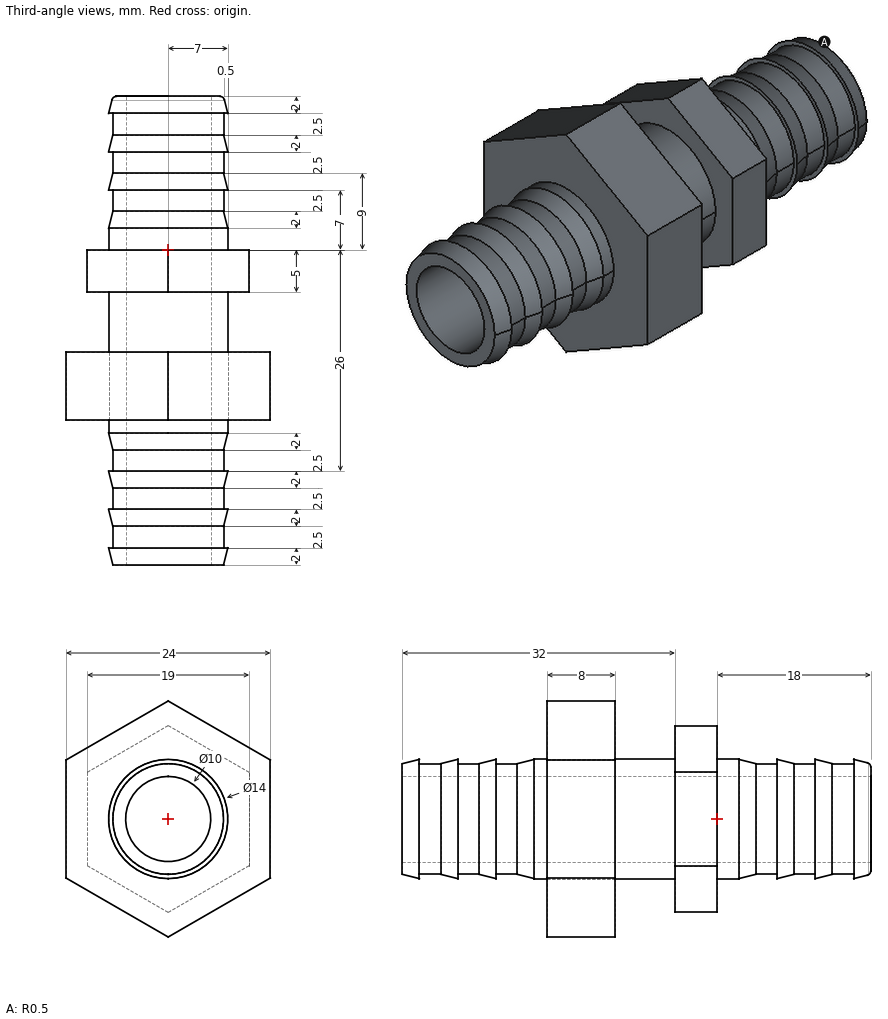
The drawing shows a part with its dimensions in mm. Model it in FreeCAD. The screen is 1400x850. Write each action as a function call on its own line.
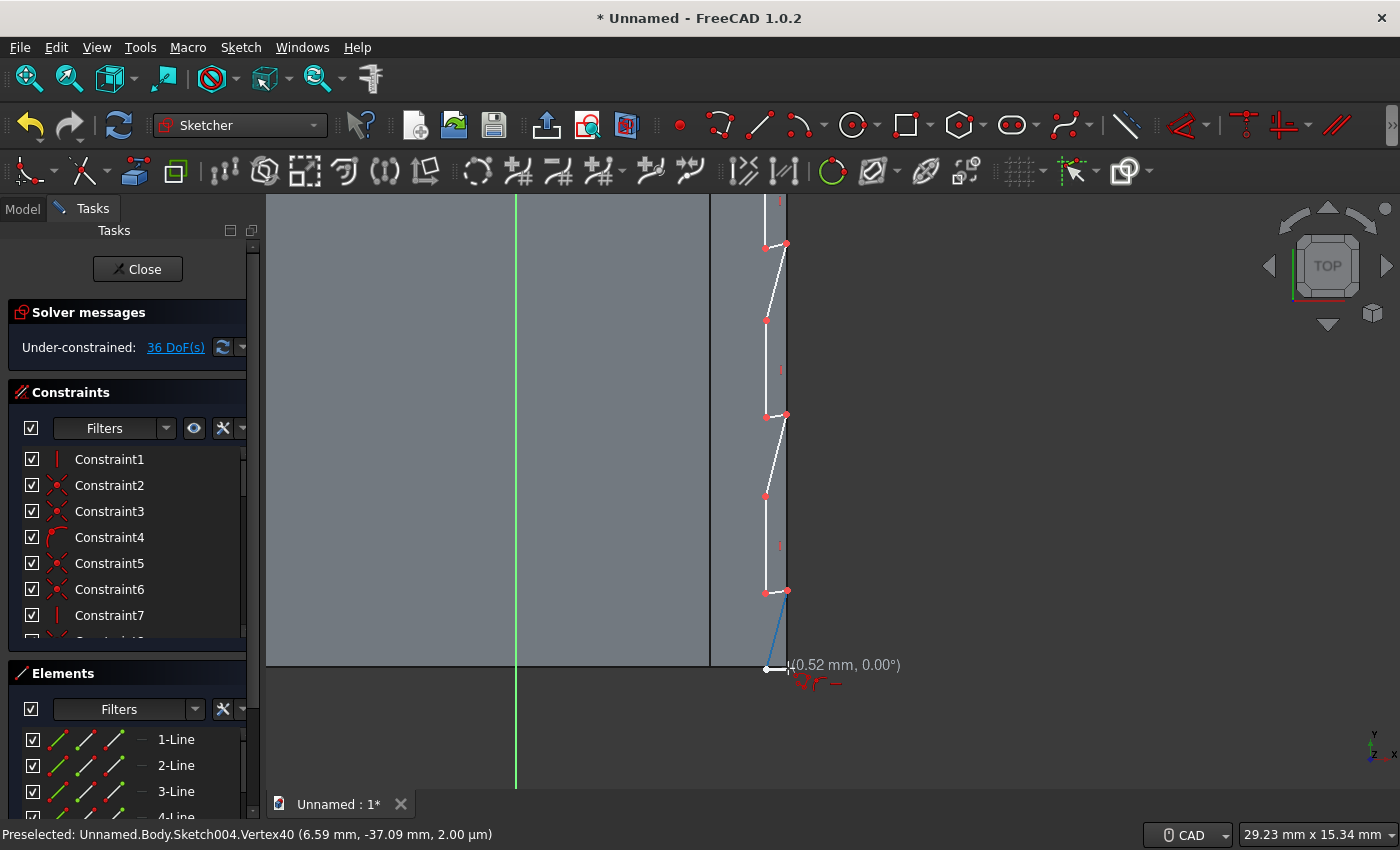
click(787, 666)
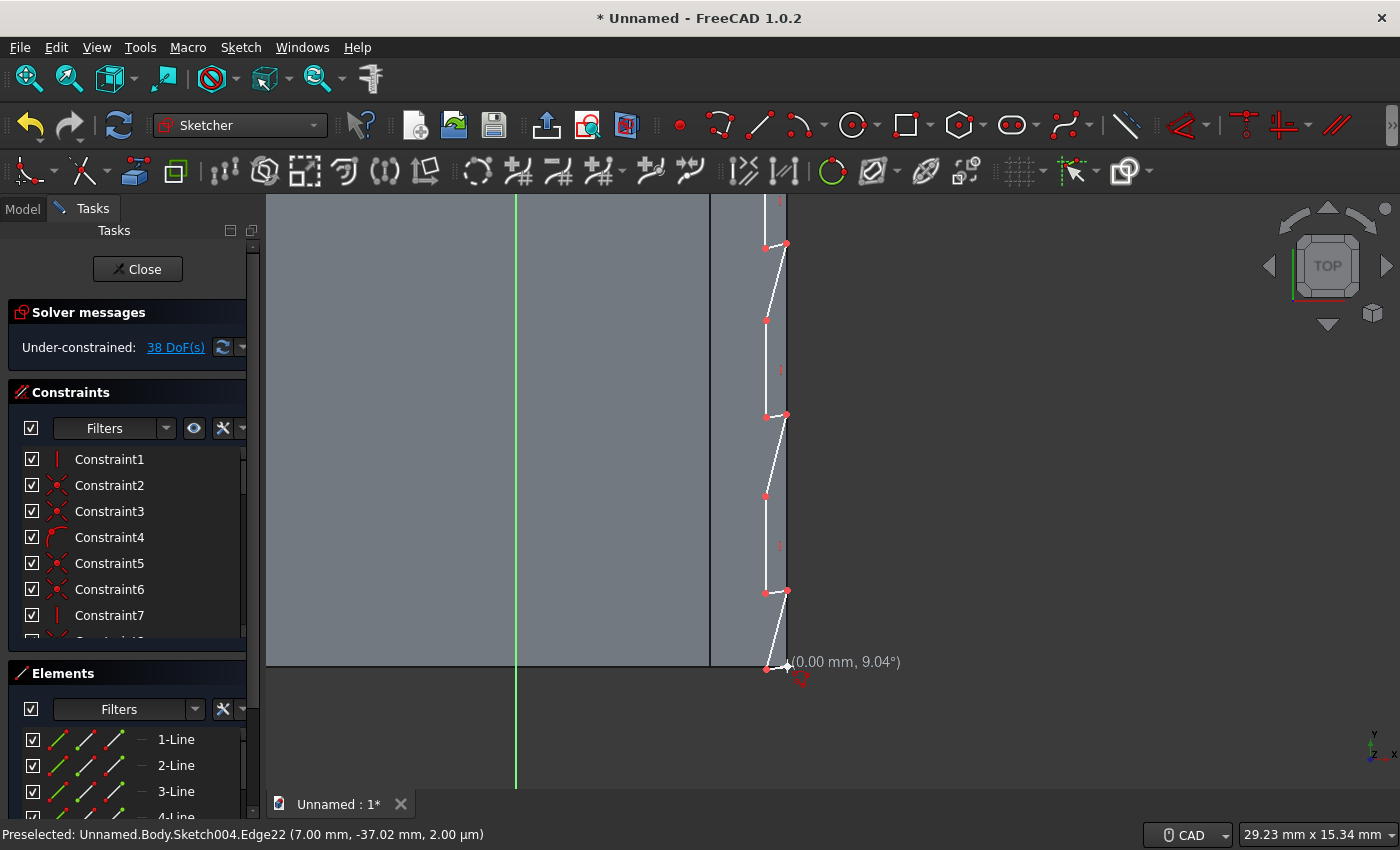
scroll(787, 668, down, 9)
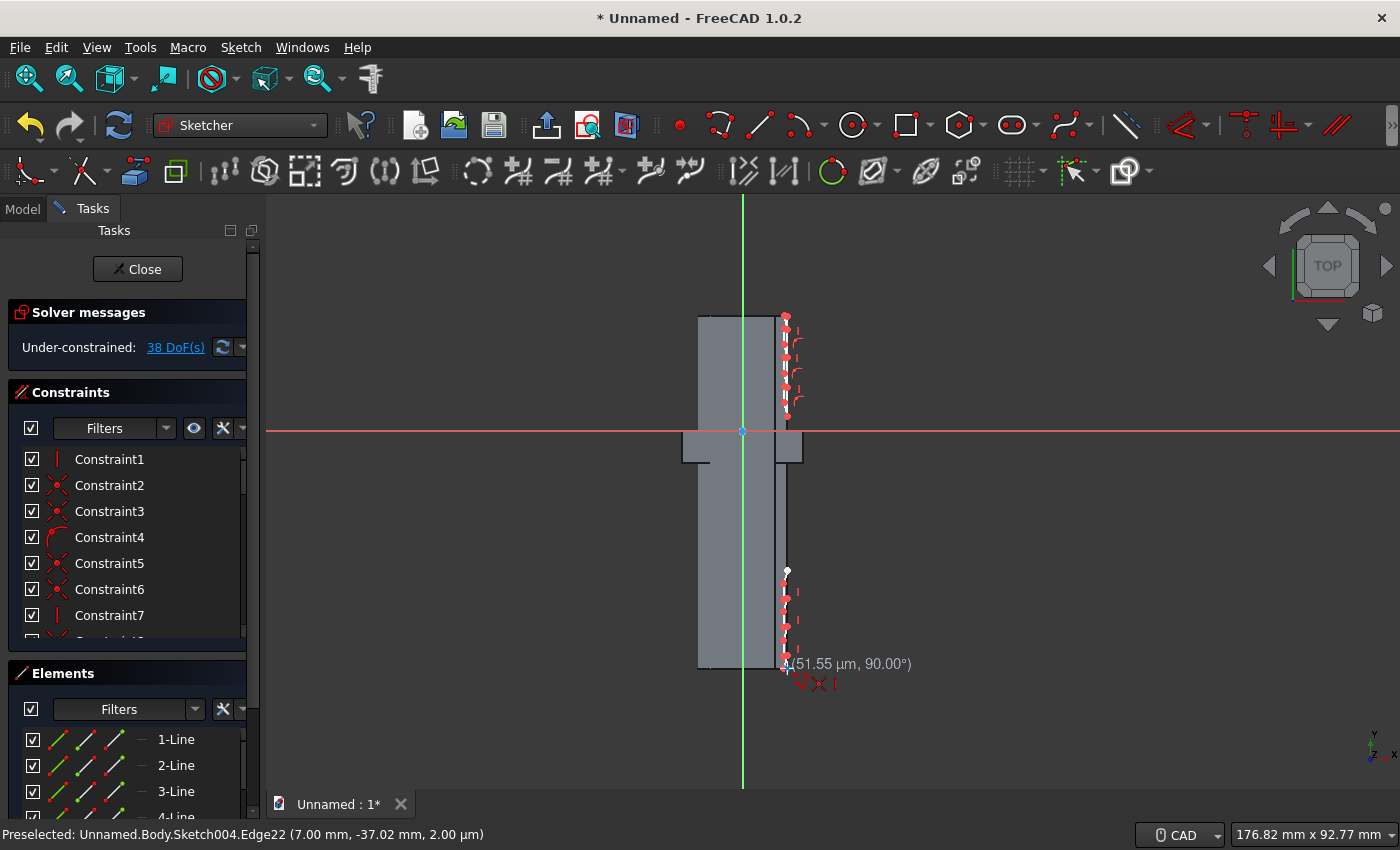
scroll(787, 569, up, 5)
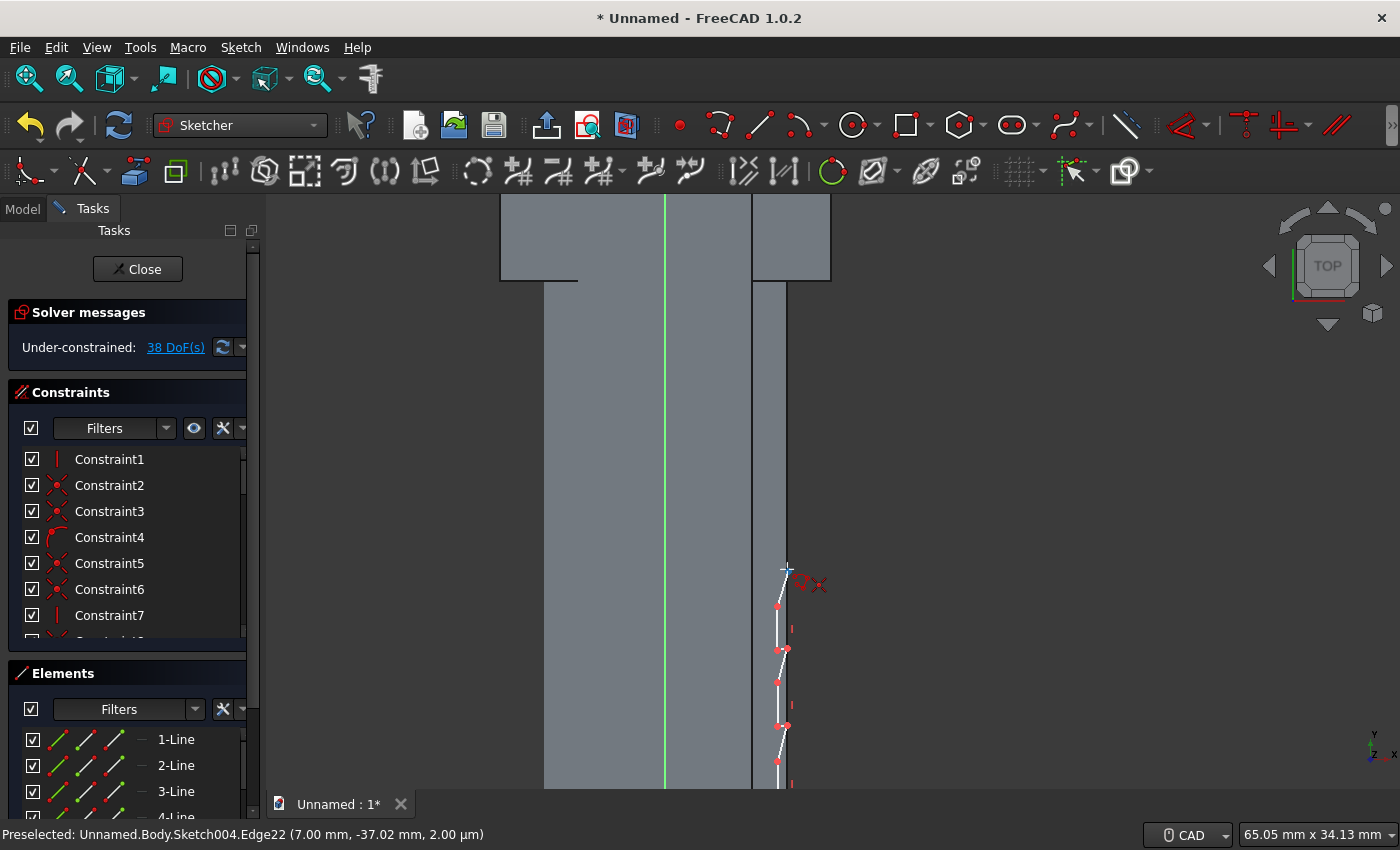
click(788, 572)
key(Escape)
key(Escape)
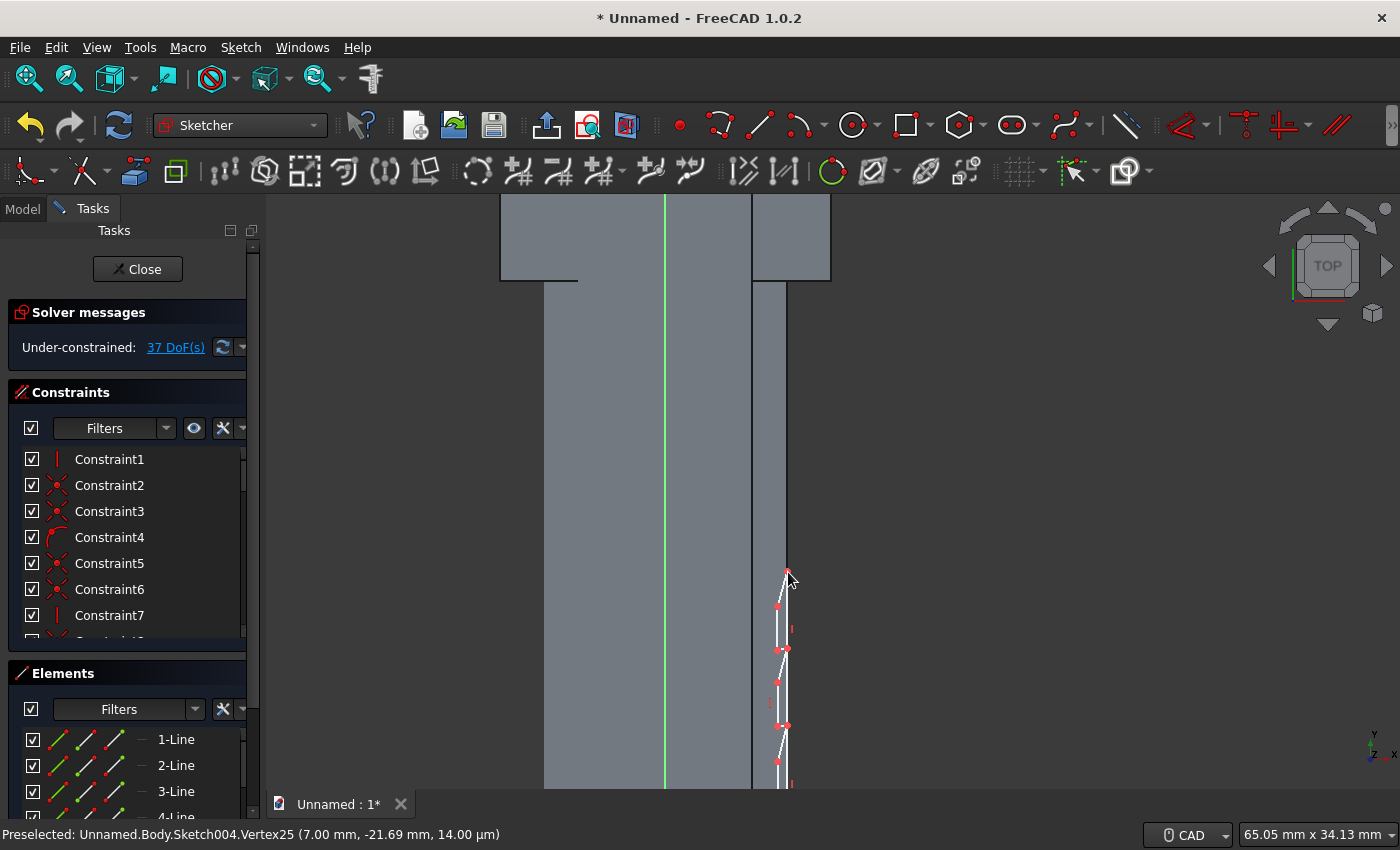
scroll(787, 569, down, 5)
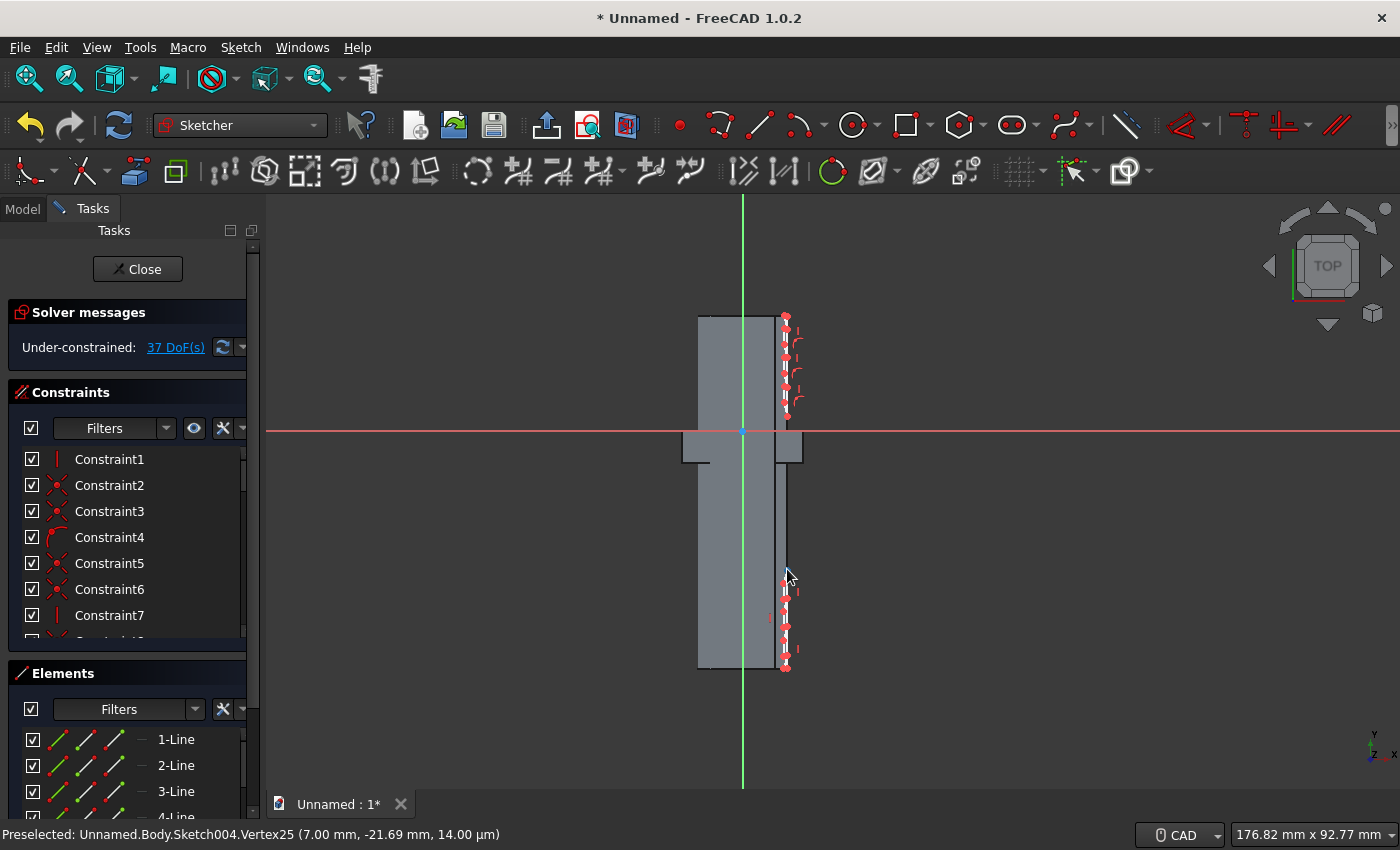
scroll(786, 316, up, 12)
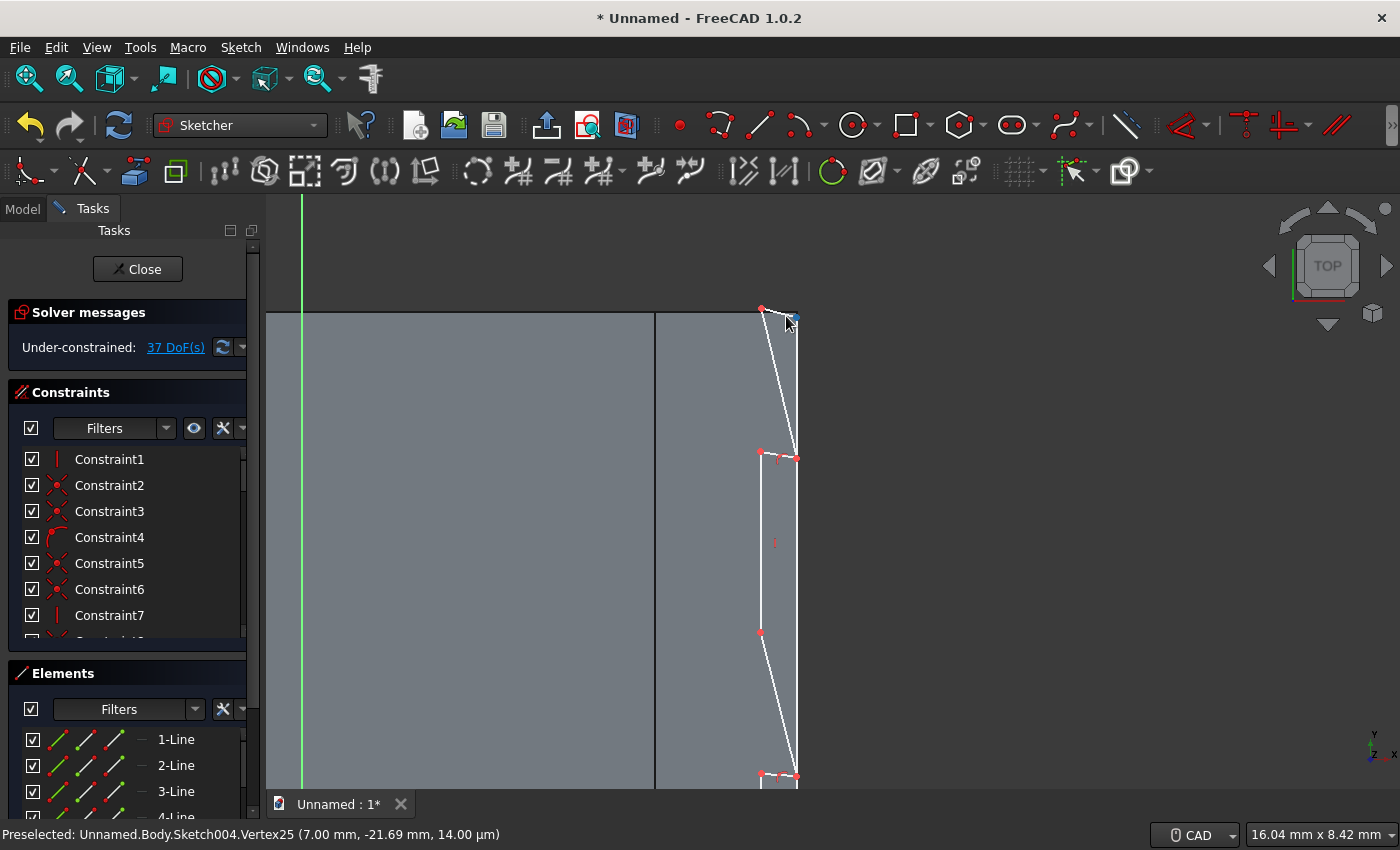
click(779, 313)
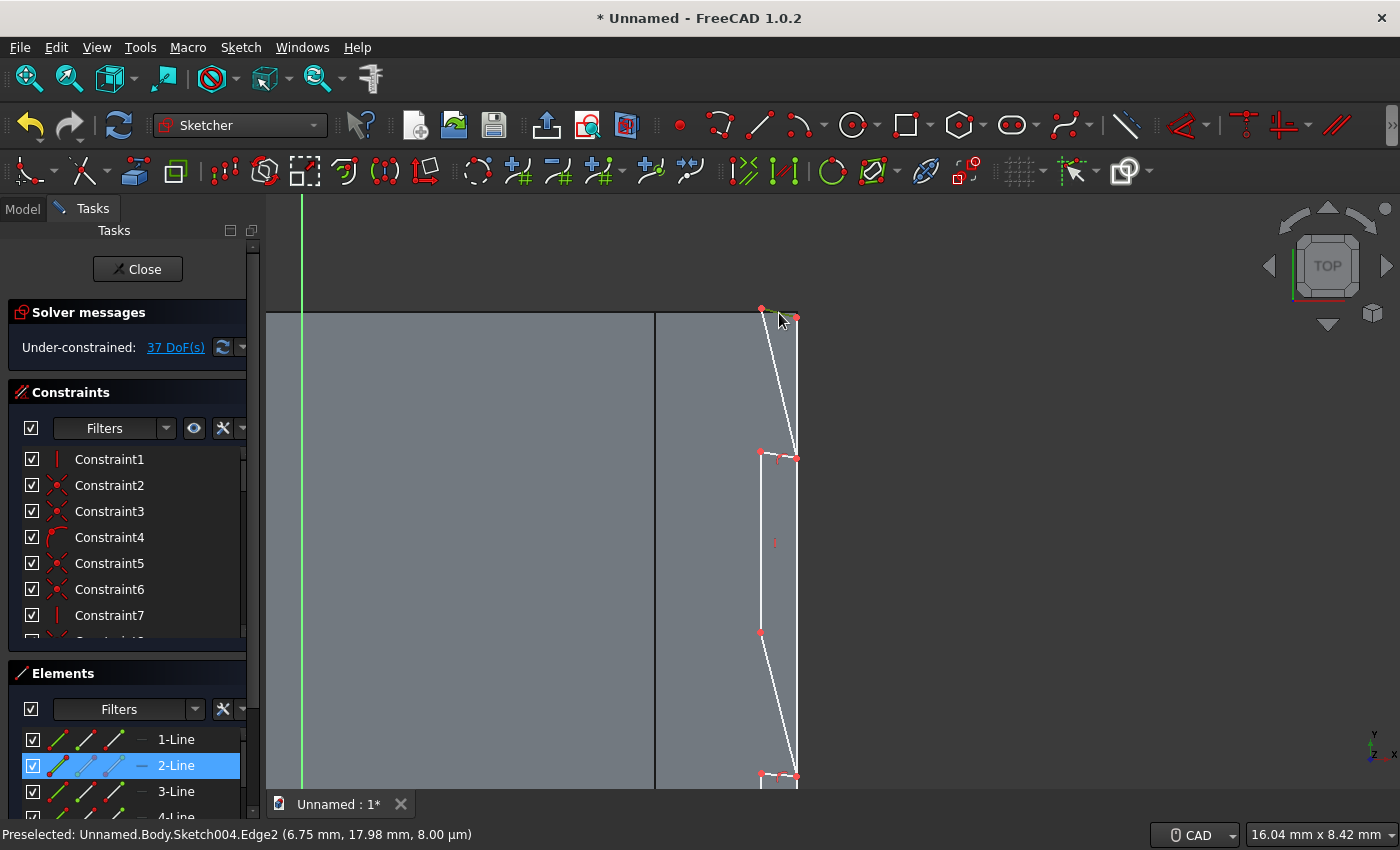
click(1310, 126)